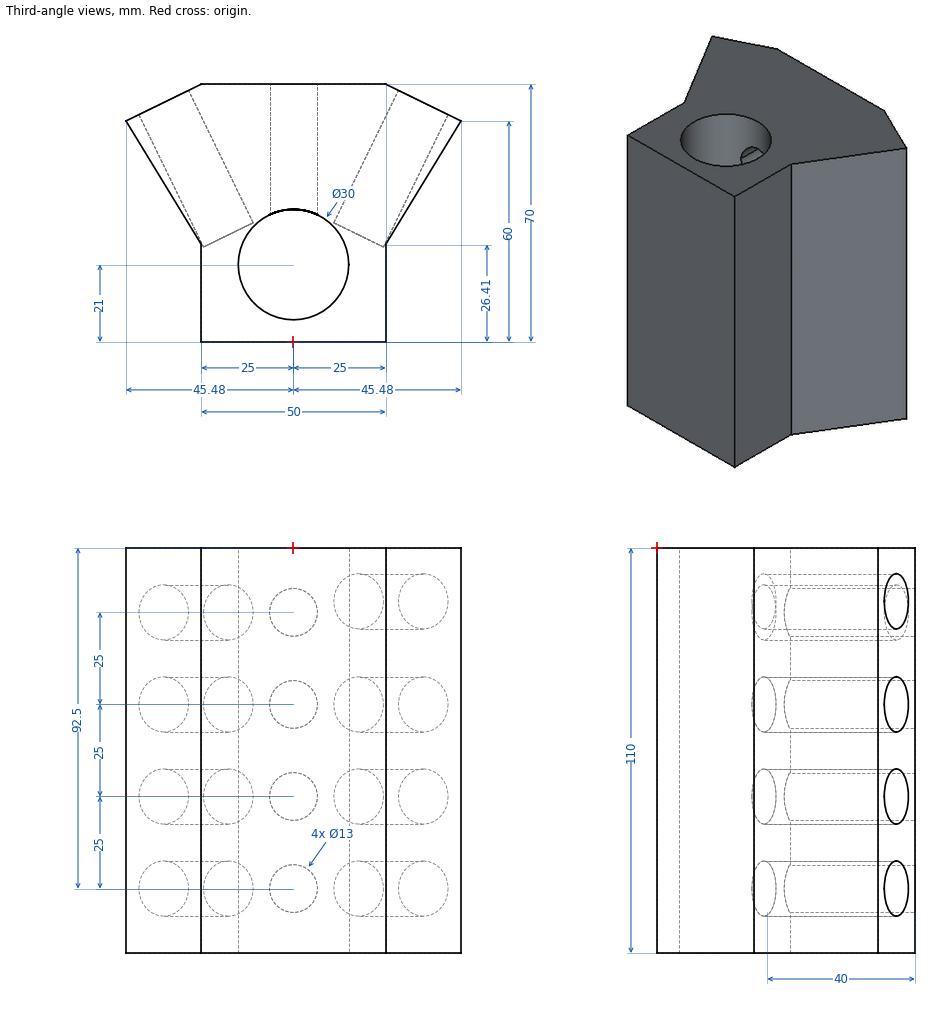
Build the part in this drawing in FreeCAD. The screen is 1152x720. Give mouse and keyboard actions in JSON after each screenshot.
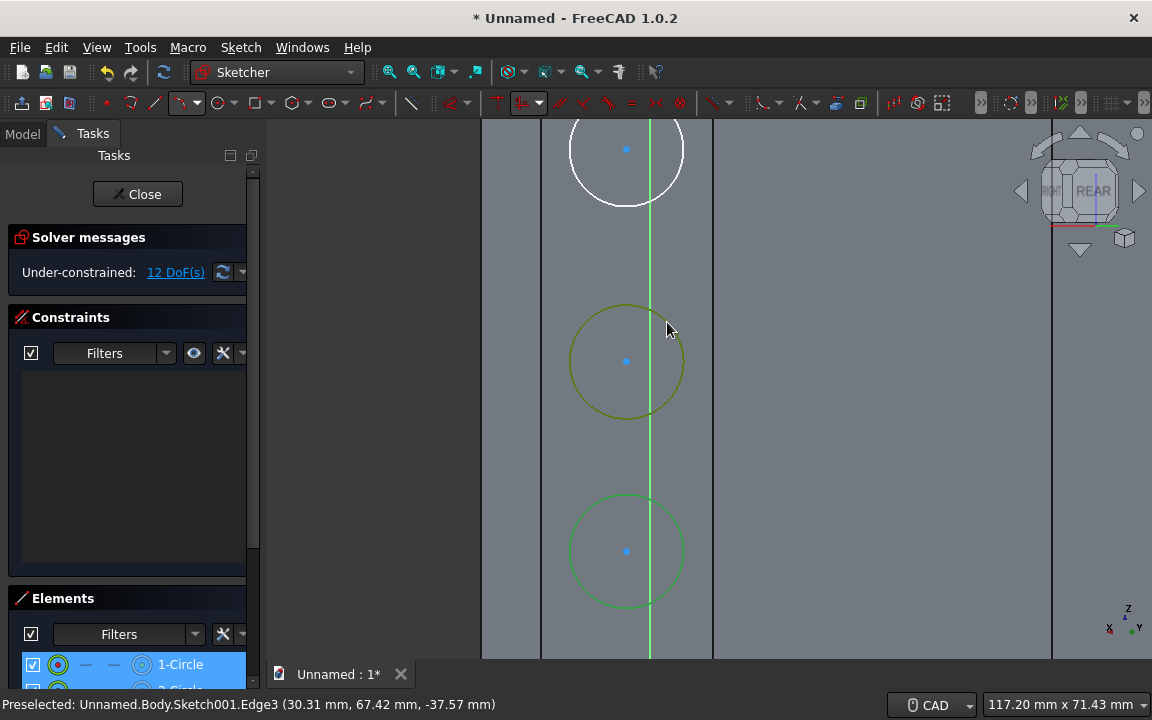
{"action": "left_click", "coordinate": [586, 190]}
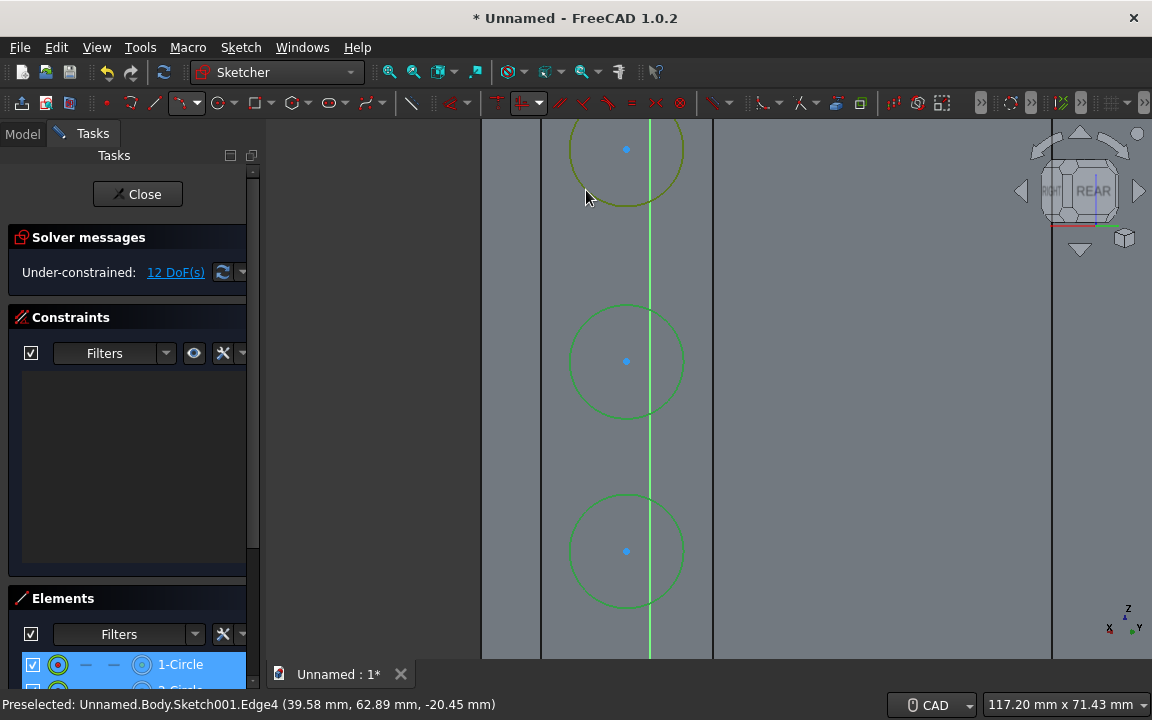
{"action": "left_click", "coordinate": [632, 104]}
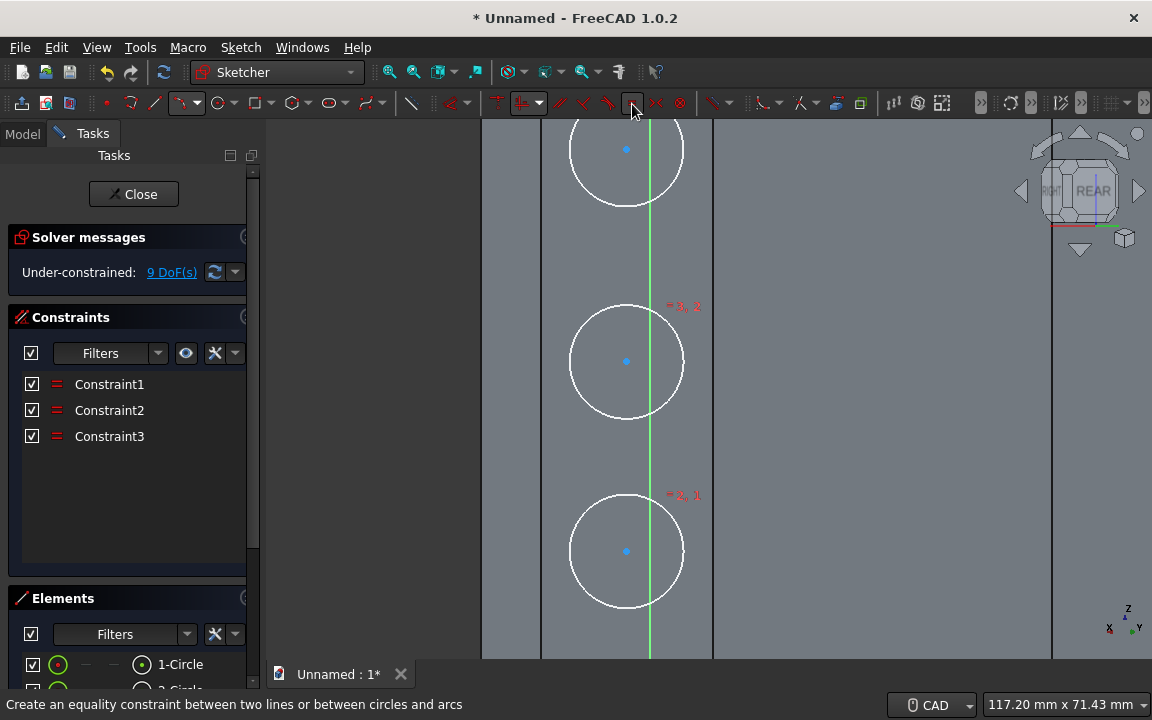
{"action": "left_click", "coordinate": [450, 104]}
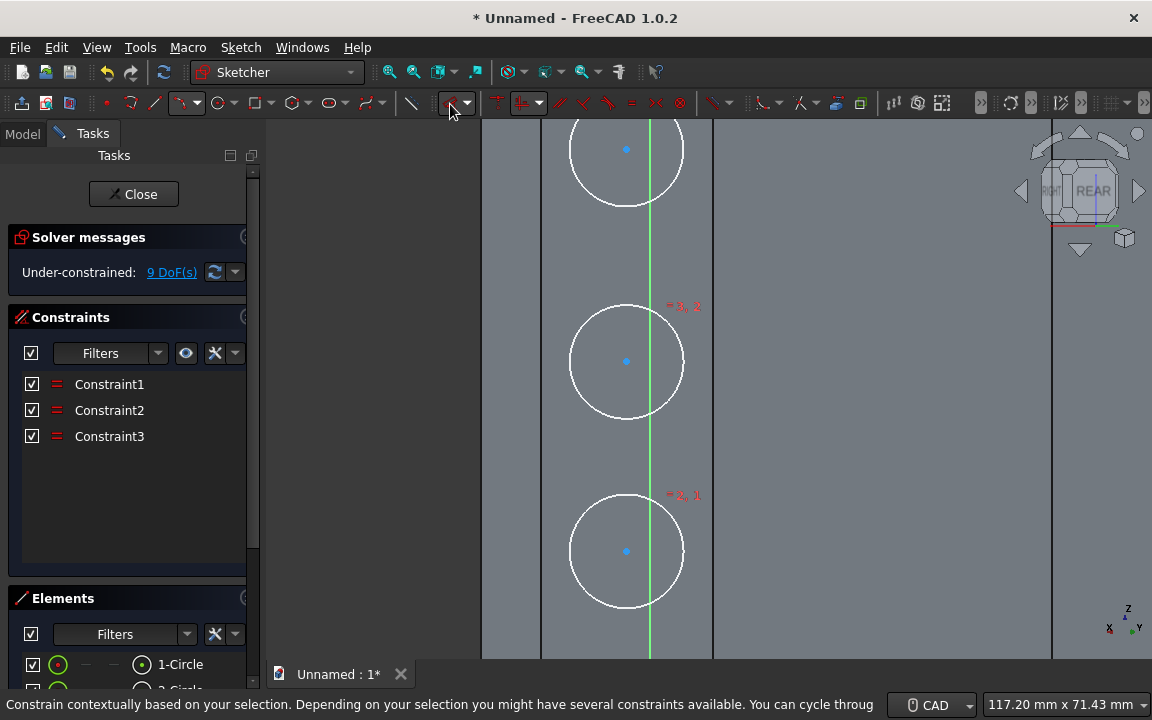
{"action": "scroll", "coordinate": [652, 366], "scroll_direction": "down", "scroll_amount": 4}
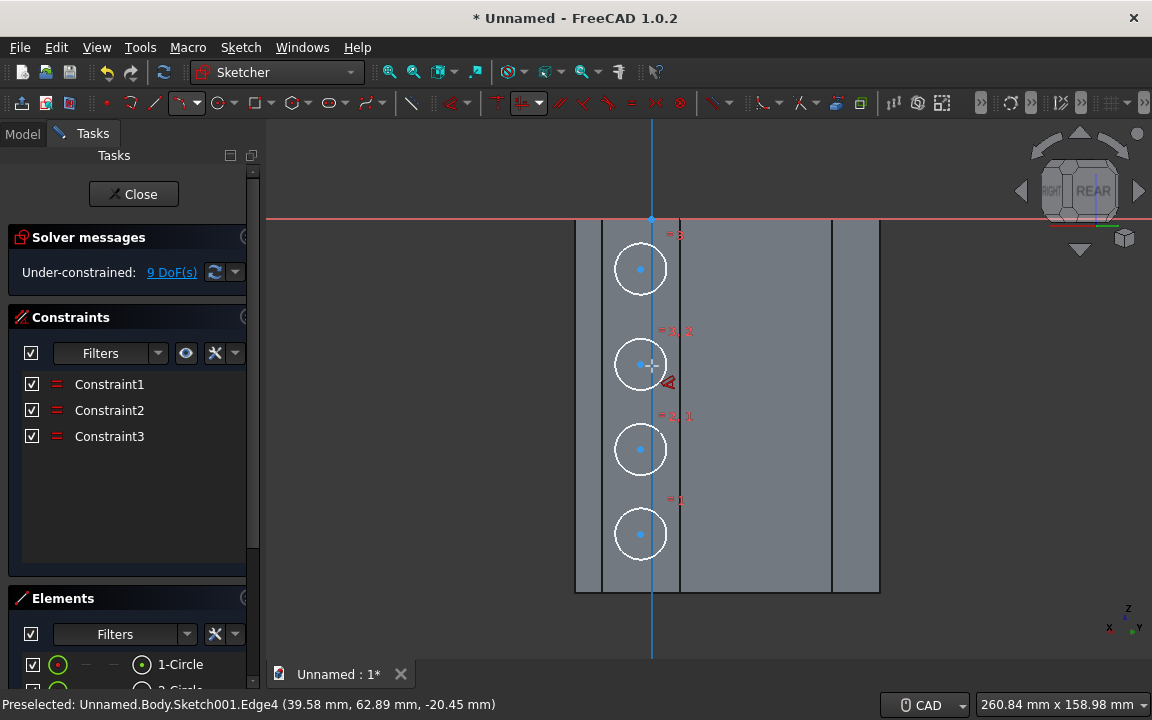
{"action": "scroll", "coordinate": [659, 516], "scroll_direction": "up", "scroll_amount": 4}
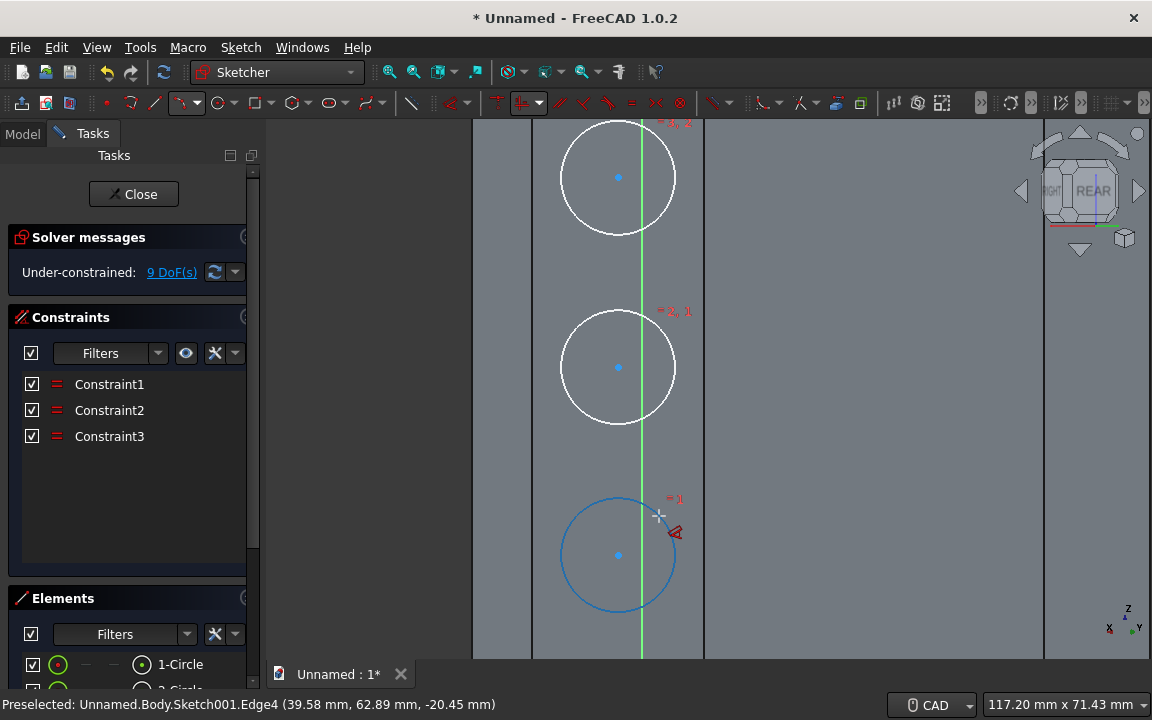
{"action": "left_click", "coordinate": [658, 515]}
{"action": "left_click", "coordinate": [681, 492]}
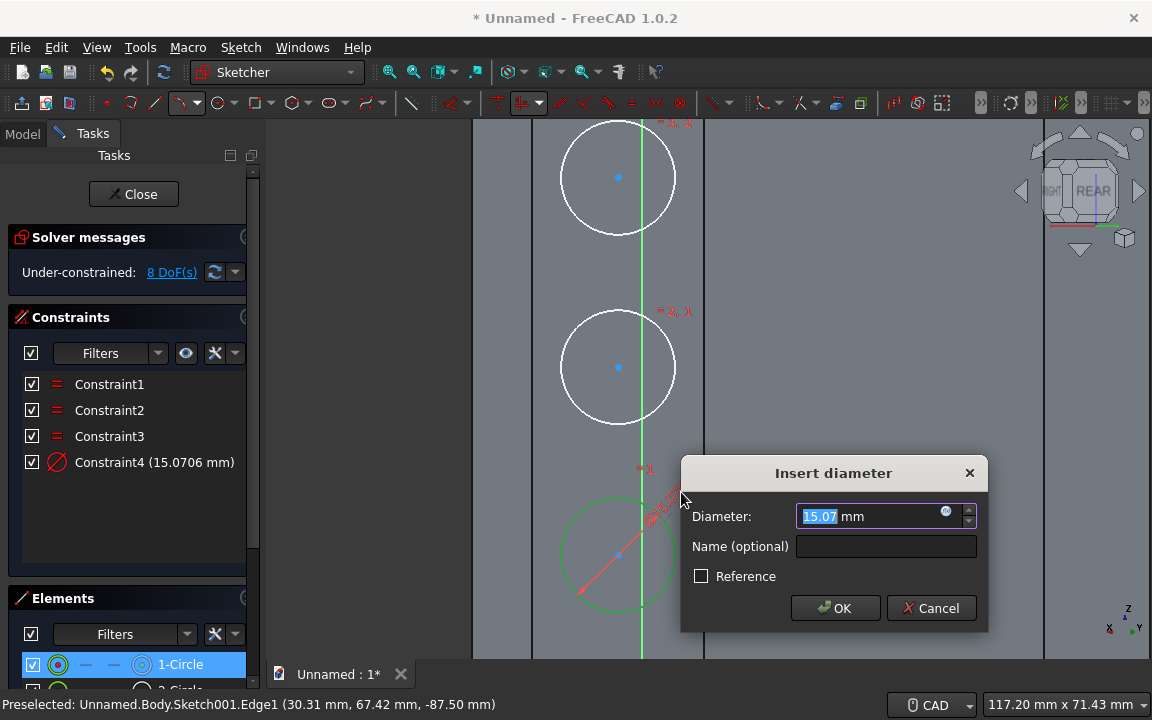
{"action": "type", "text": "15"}
{"action": "key", "text": "Return"}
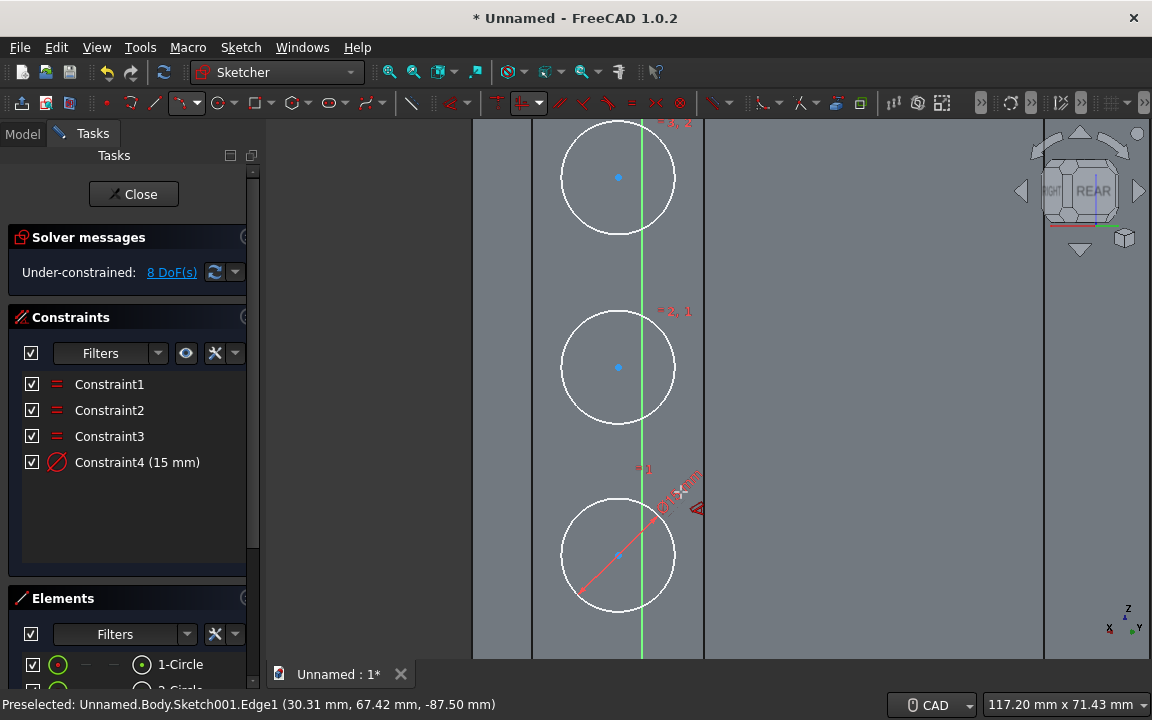
{"action": "left_click", "coordinate": [618, 555]}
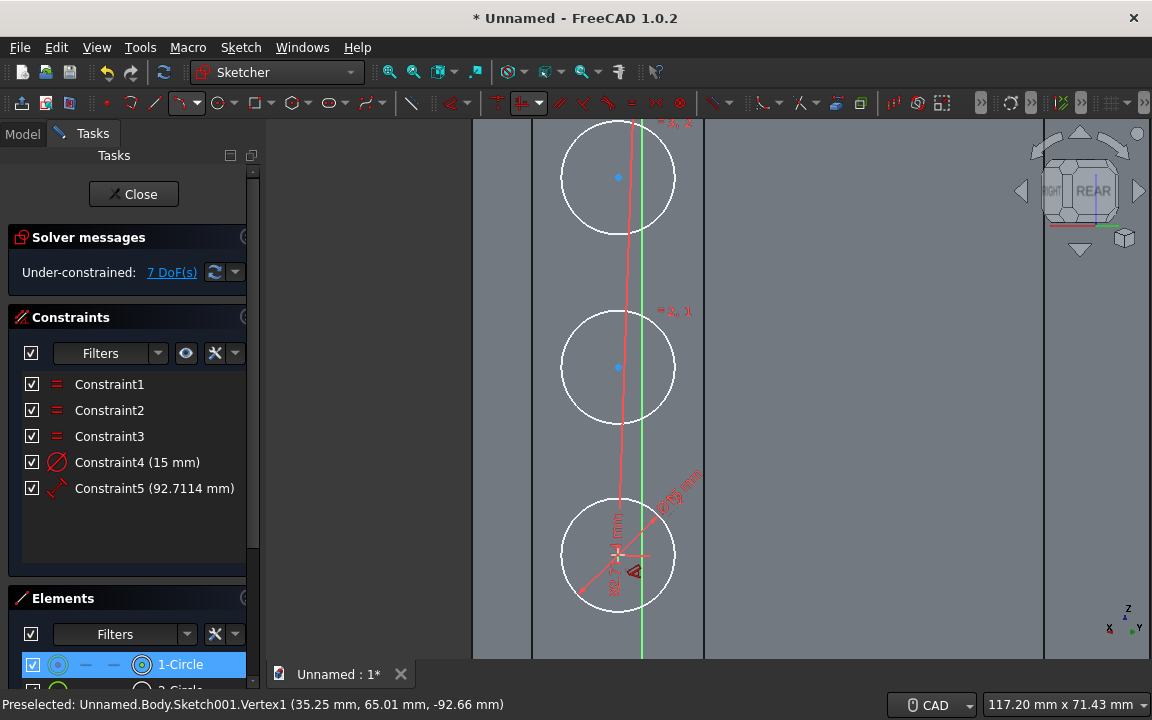
{"action": "left_click", "coordinate": [618, 367]}
{"action": "left_click", "coordinate": [584, 461]}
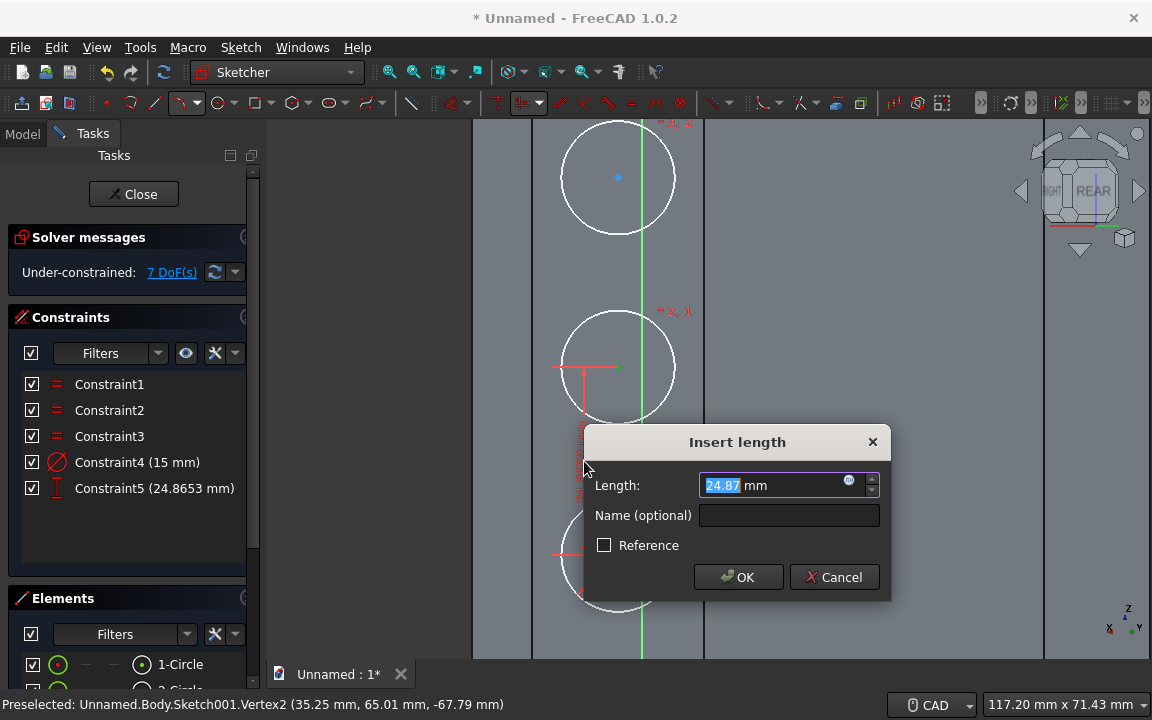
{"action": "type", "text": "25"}
{"action": "key", "text": "Return"}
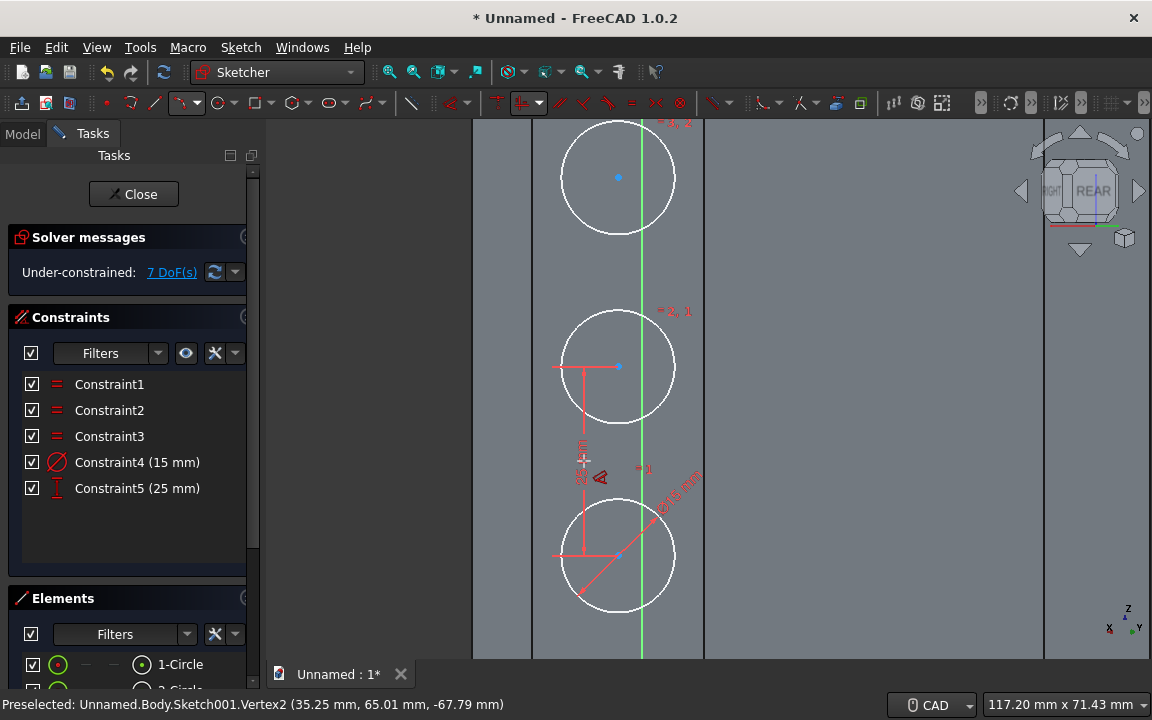
{"action": "left_click", "coordinate": [618, 367]}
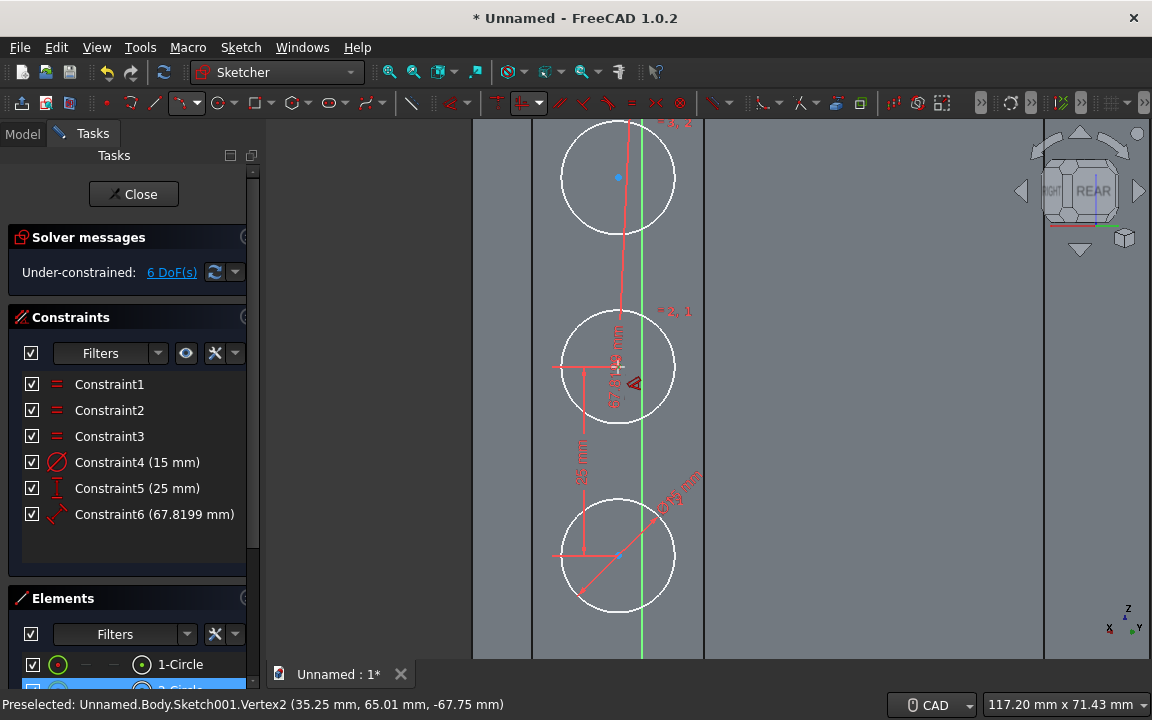
{"action": "left_click", "coordinate": [618, 178]}
{"action": "left_click", "coordinate": [584, 272]}